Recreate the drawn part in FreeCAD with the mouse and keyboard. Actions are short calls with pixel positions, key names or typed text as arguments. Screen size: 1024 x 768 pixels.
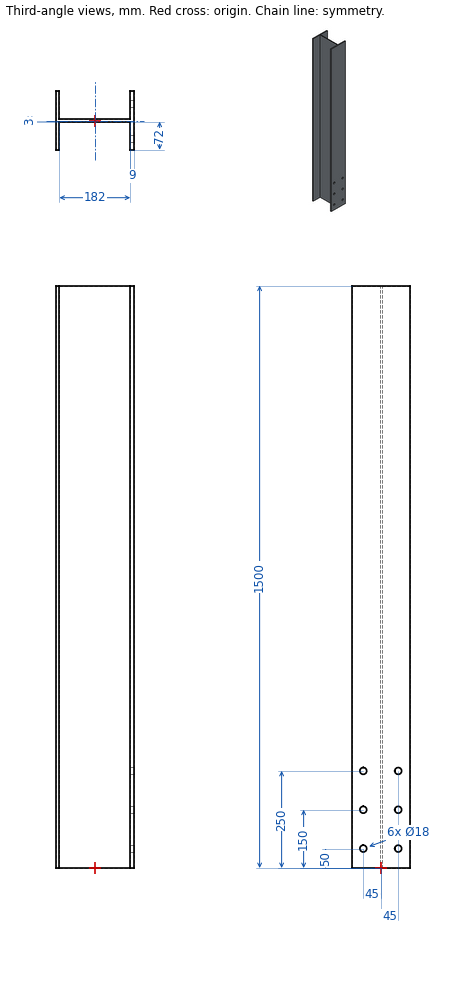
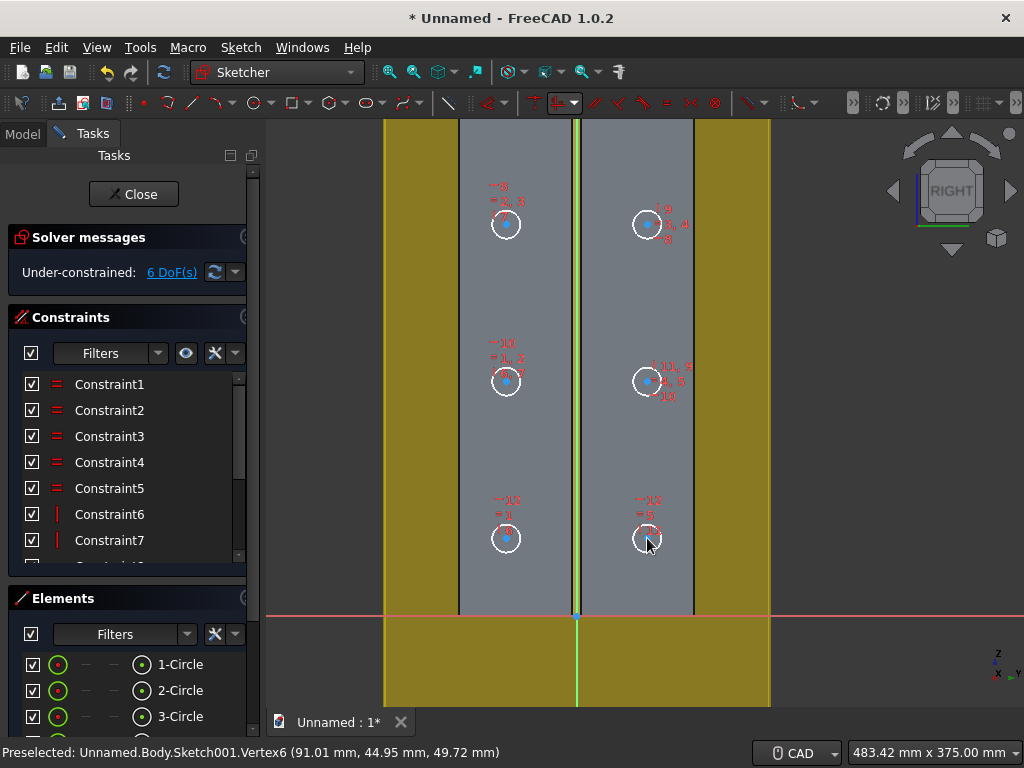
click(488, 104)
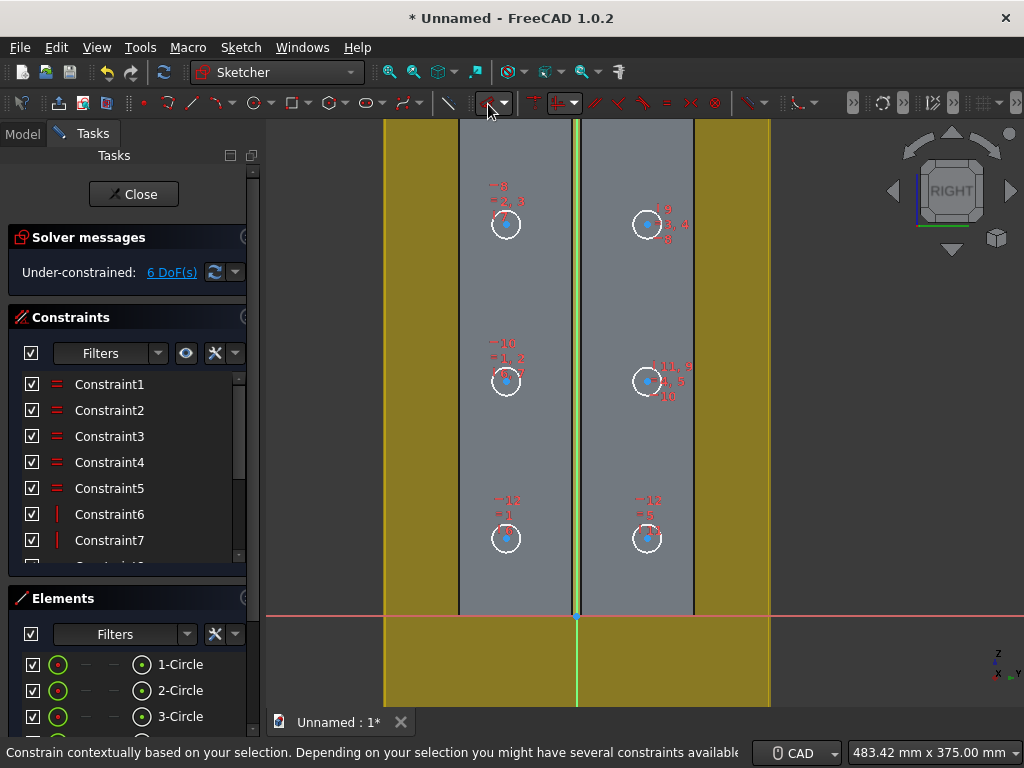
scroll(516, 529, up, 2)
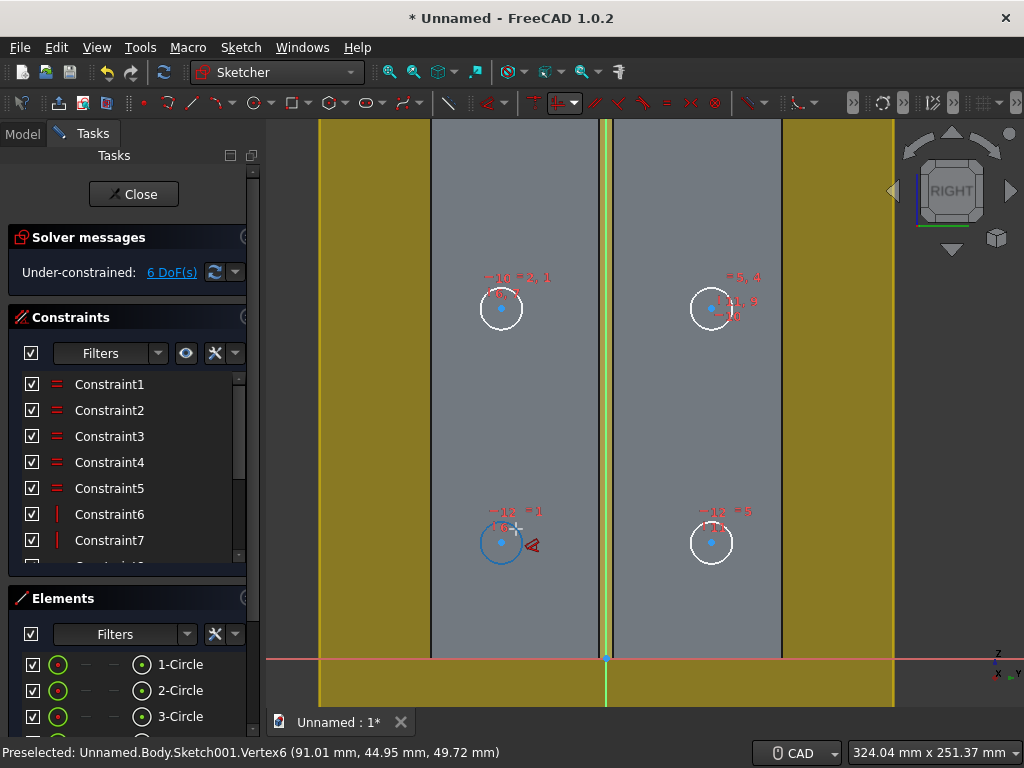
click(516, 528)
click(538, 505)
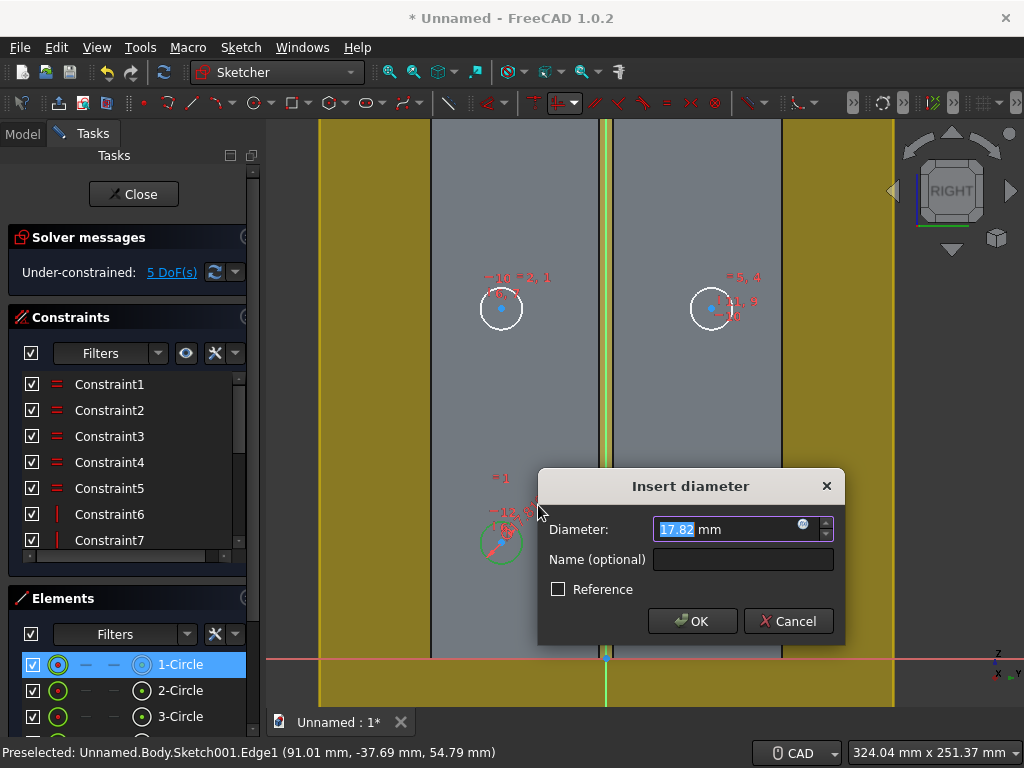
text(18)
key(Return)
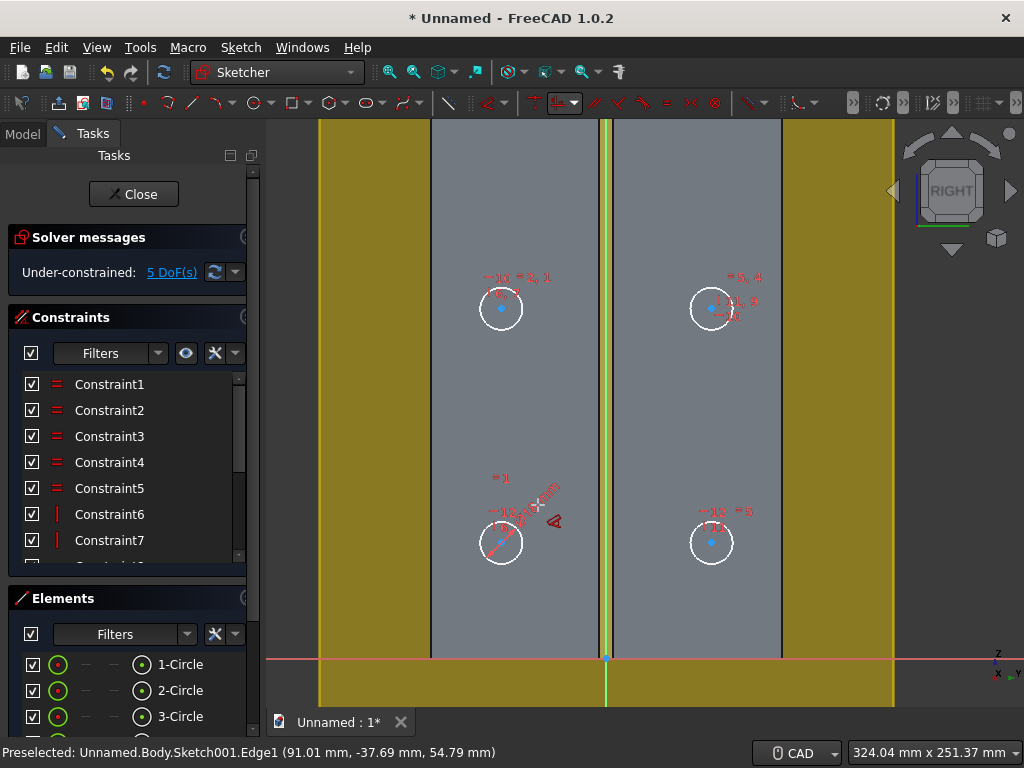
click(501, 543)
click(554, 485)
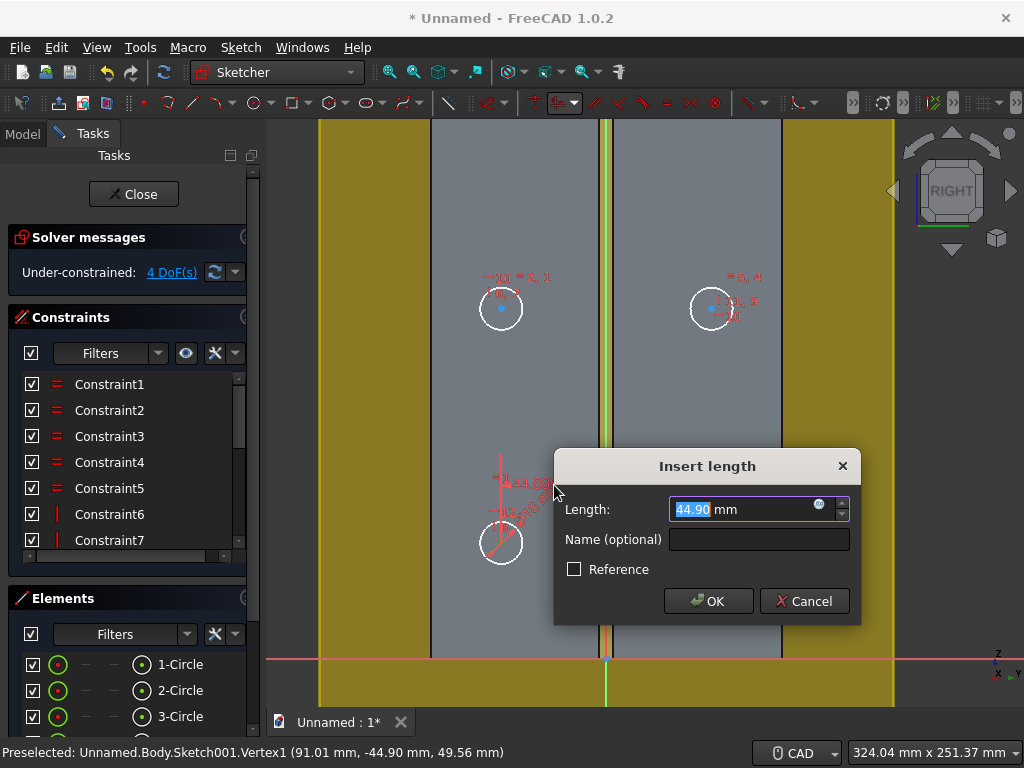
text(45)
key(Return)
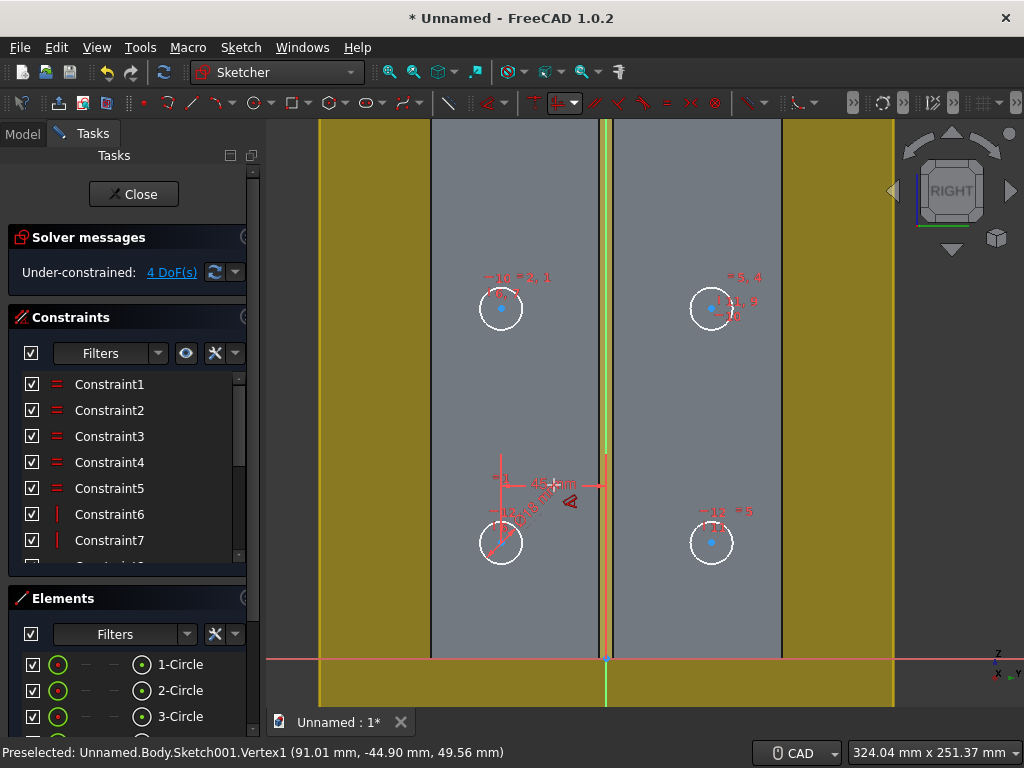
click(501, 543)
click(467, 601)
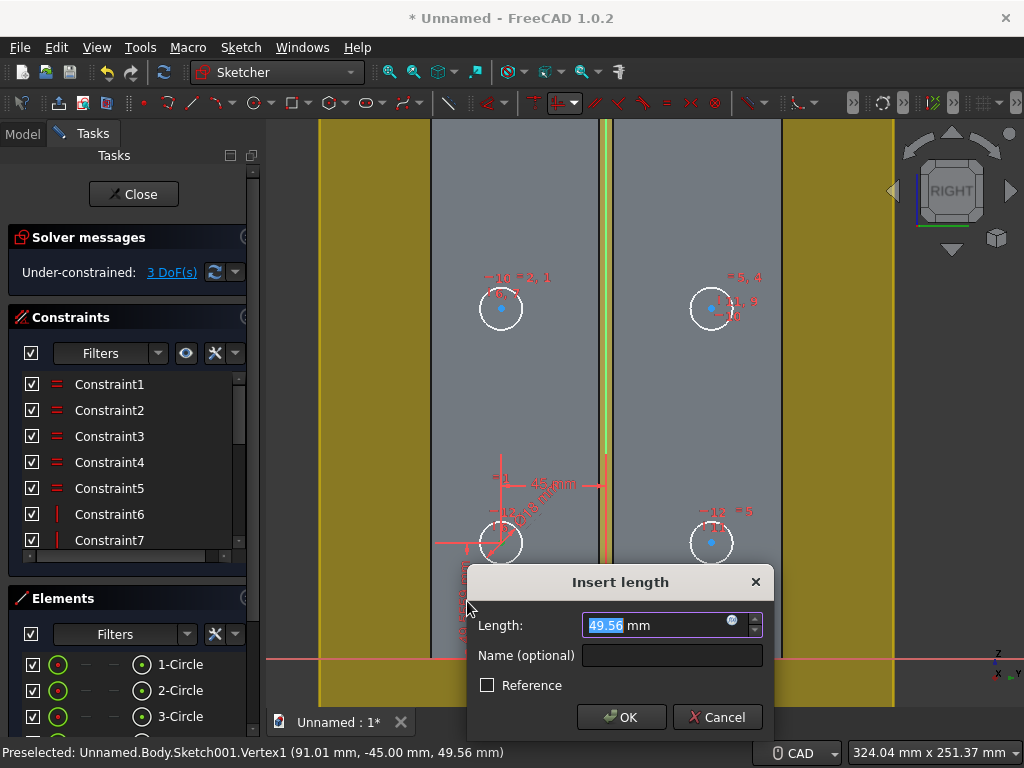
text(50)
key(Return)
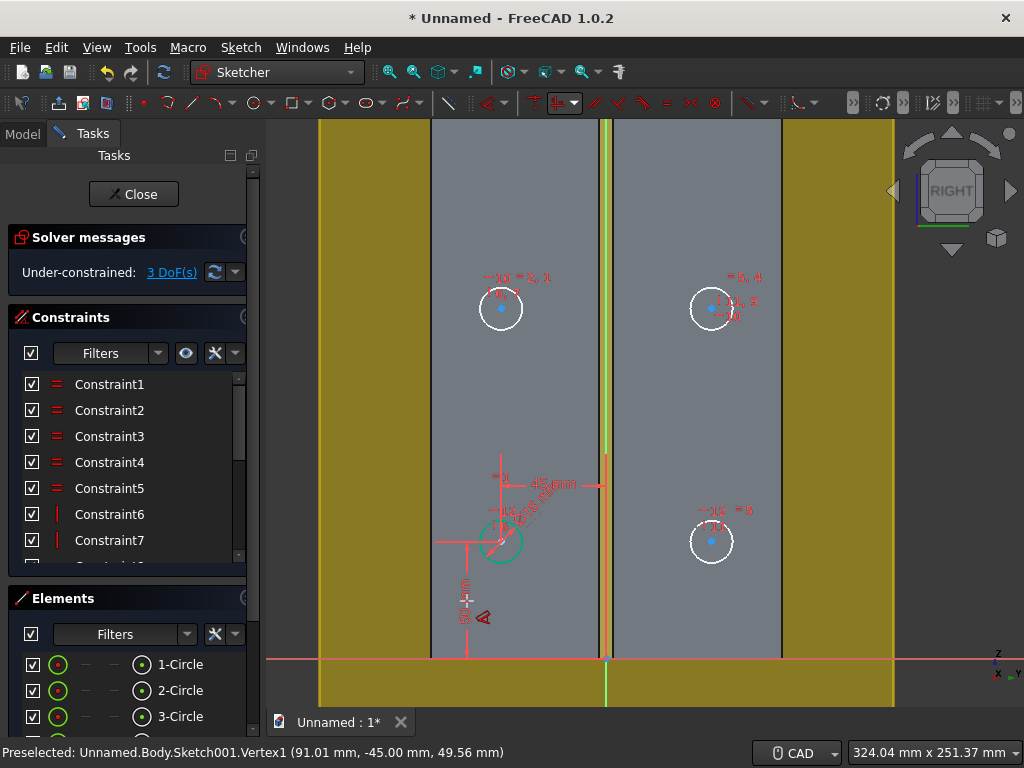
scroll(516, 529, down, 2)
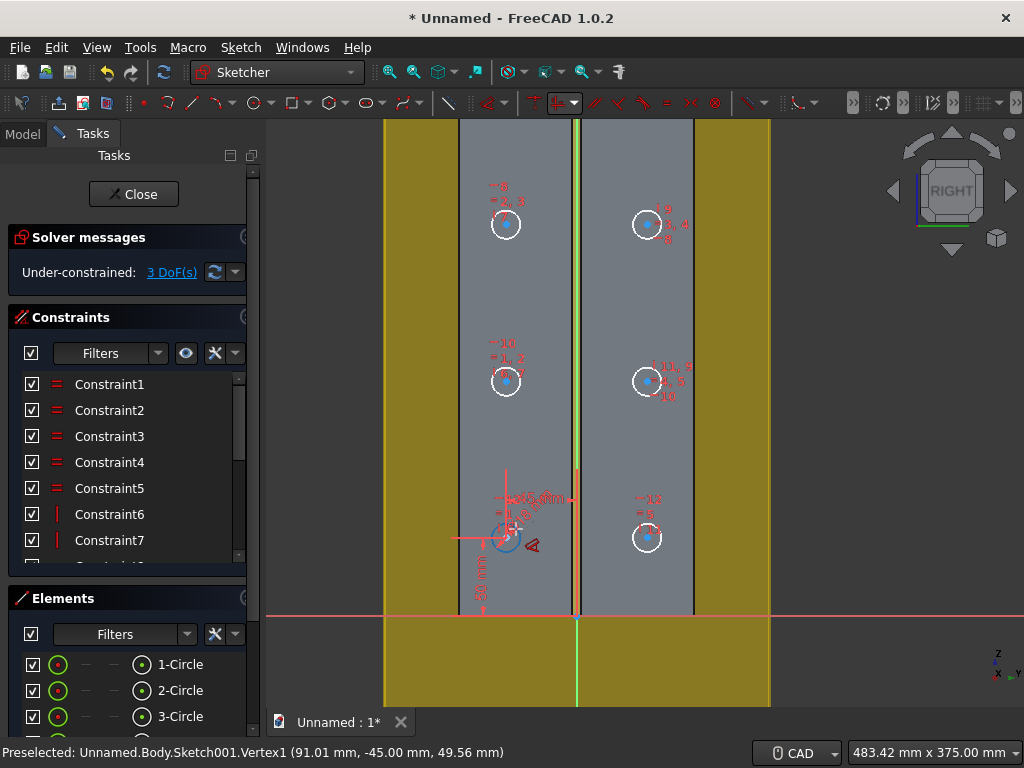
click(647, 225)
click(612, 650)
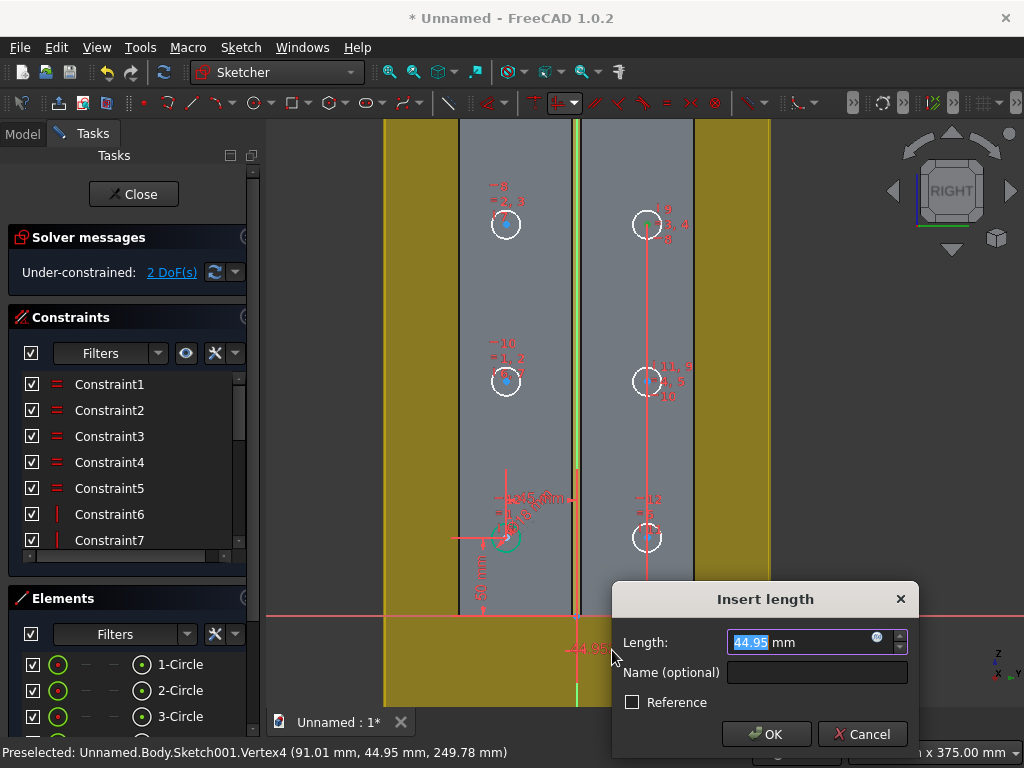
text(45)
key(Return)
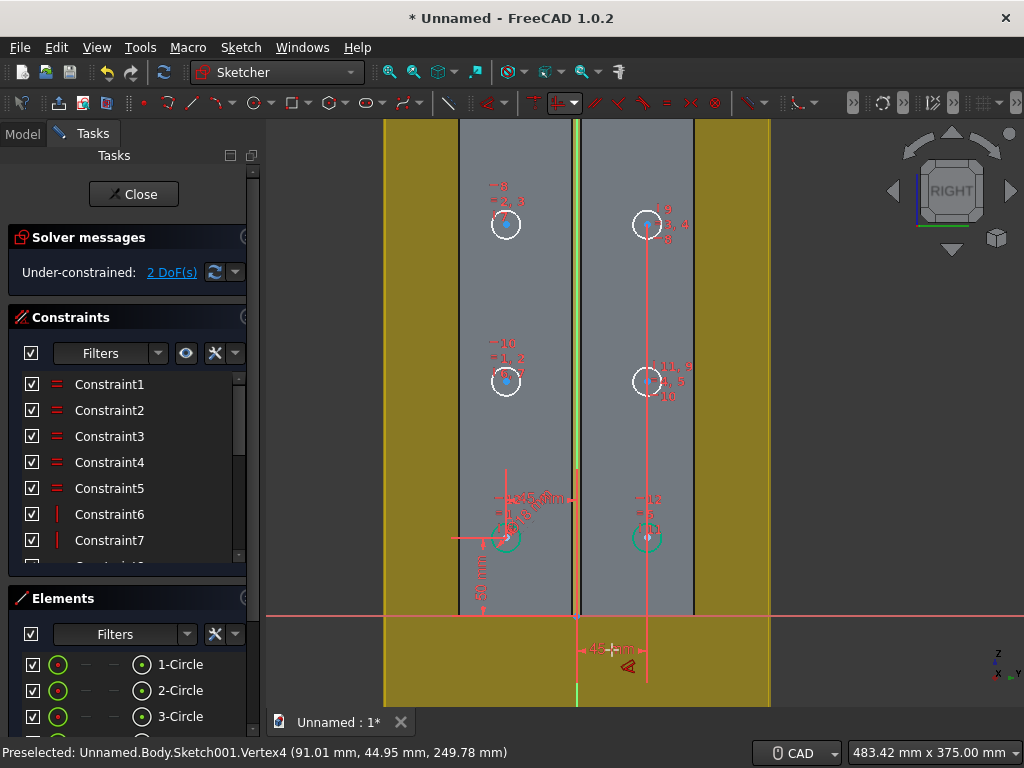
click(506, 382)
click(472, 445)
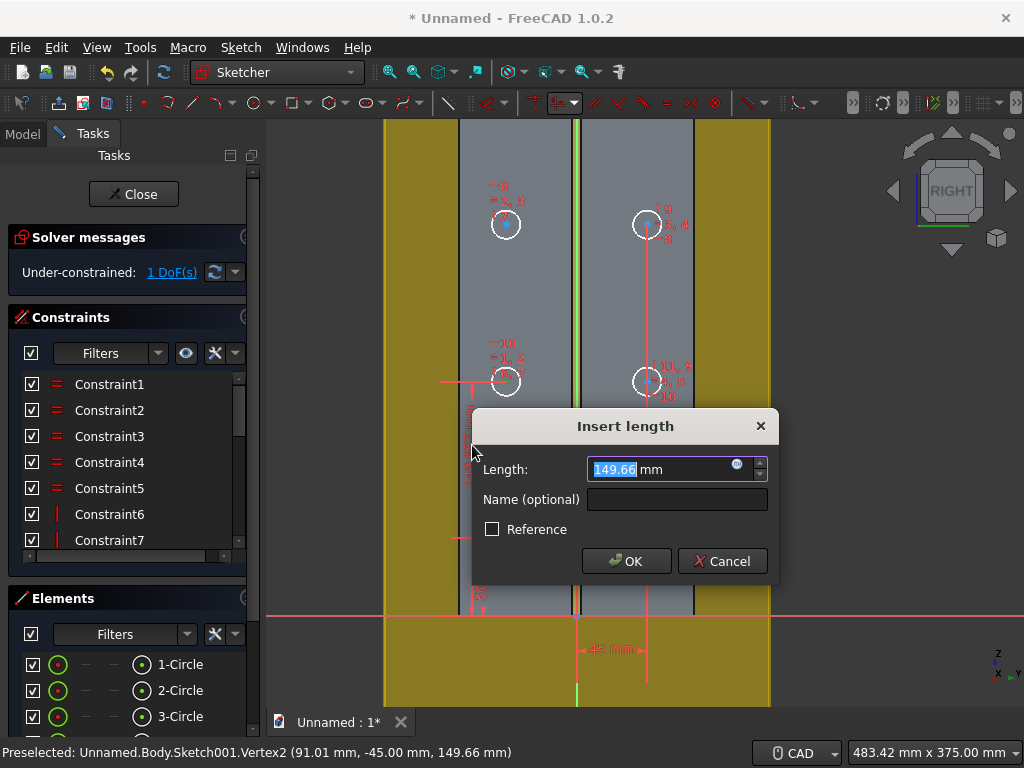
text(150)
key(Return)